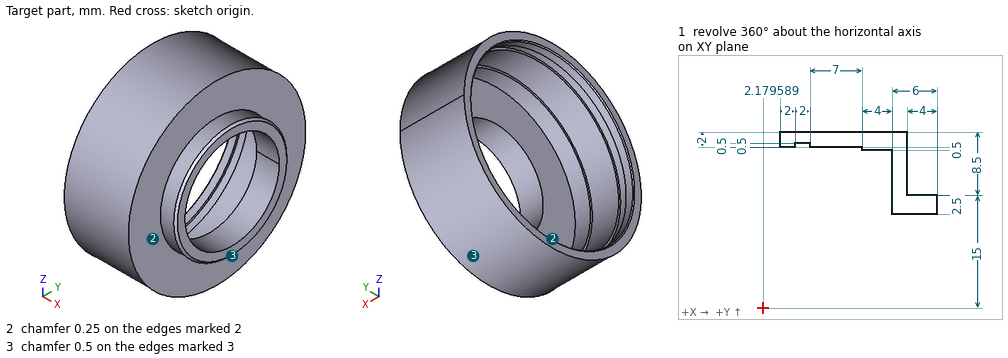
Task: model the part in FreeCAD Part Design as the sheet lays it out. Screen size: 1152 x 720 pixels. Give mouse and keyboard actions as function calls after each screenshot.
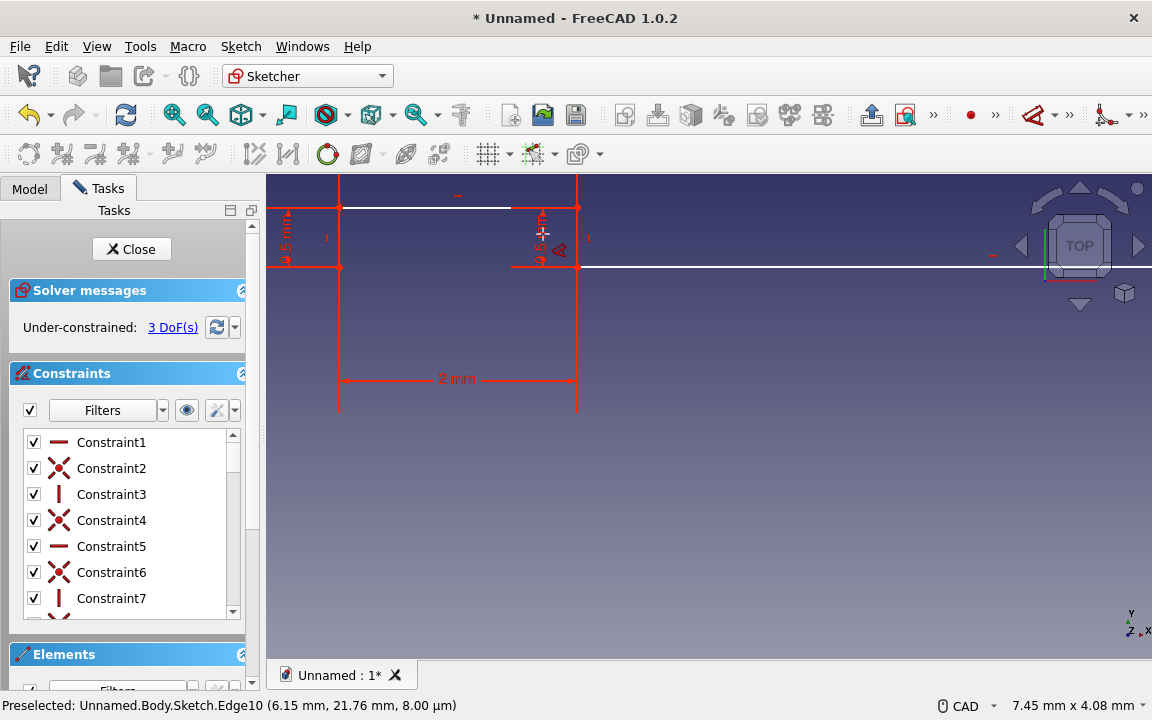
scroll(568, 292, down, 11)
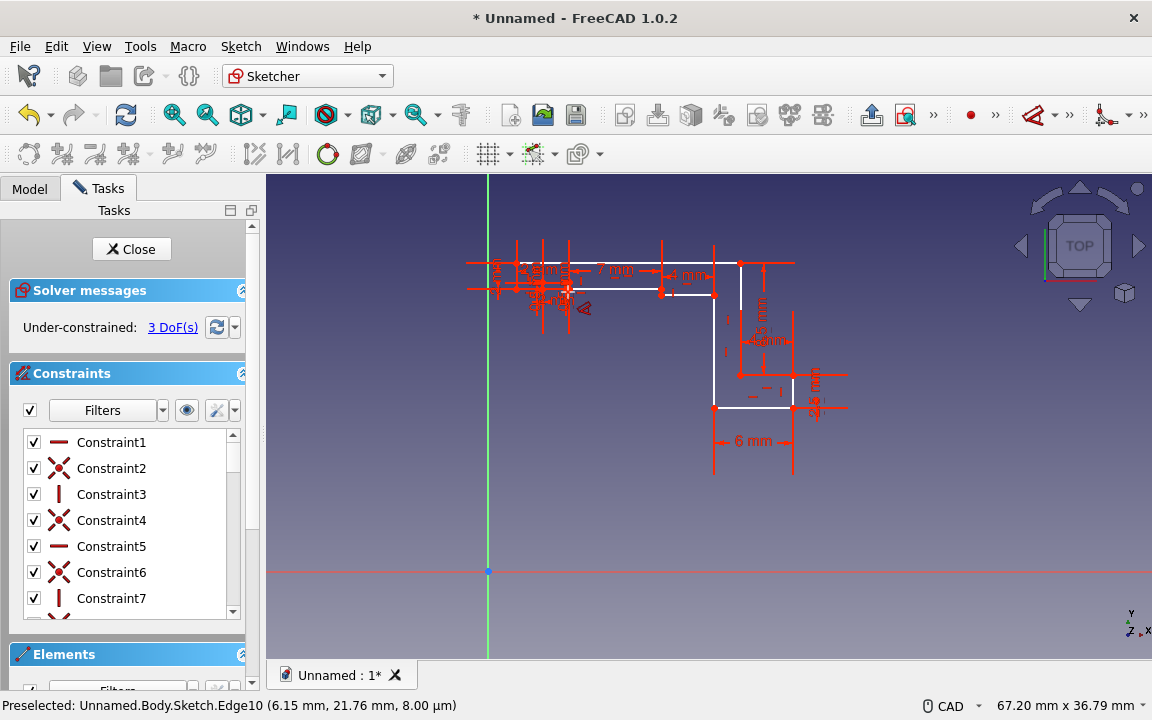
scroll(662, 291, up, 11)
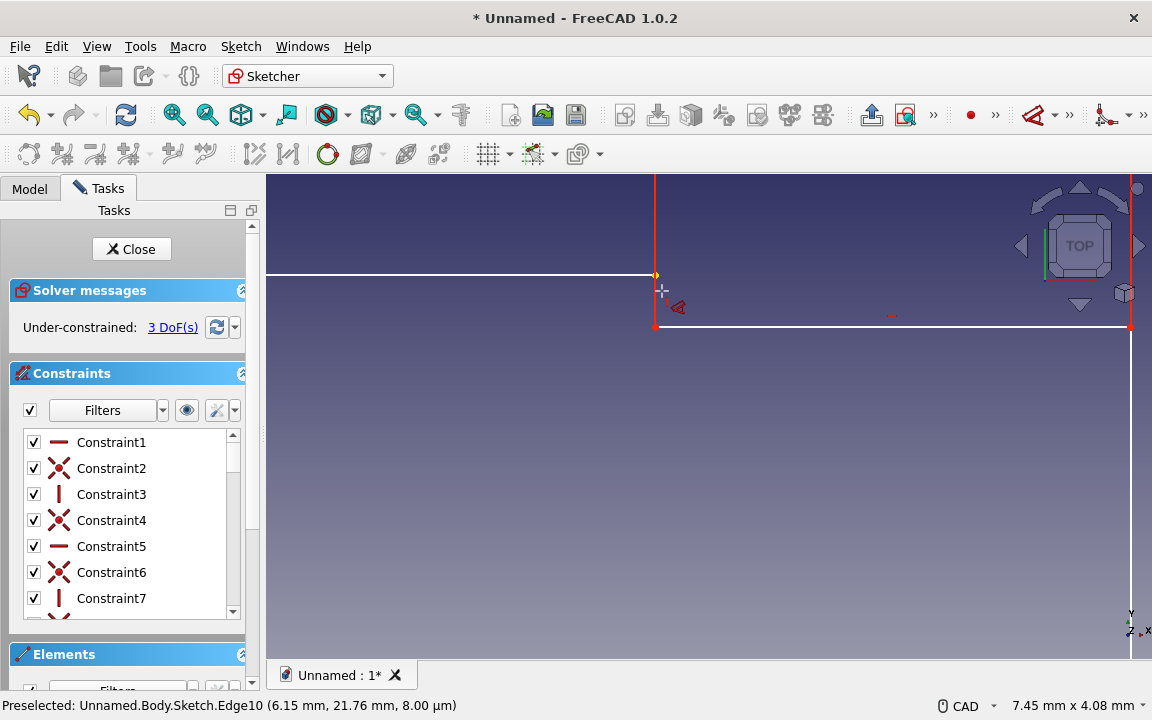
click(655, 291)
click(689, 301)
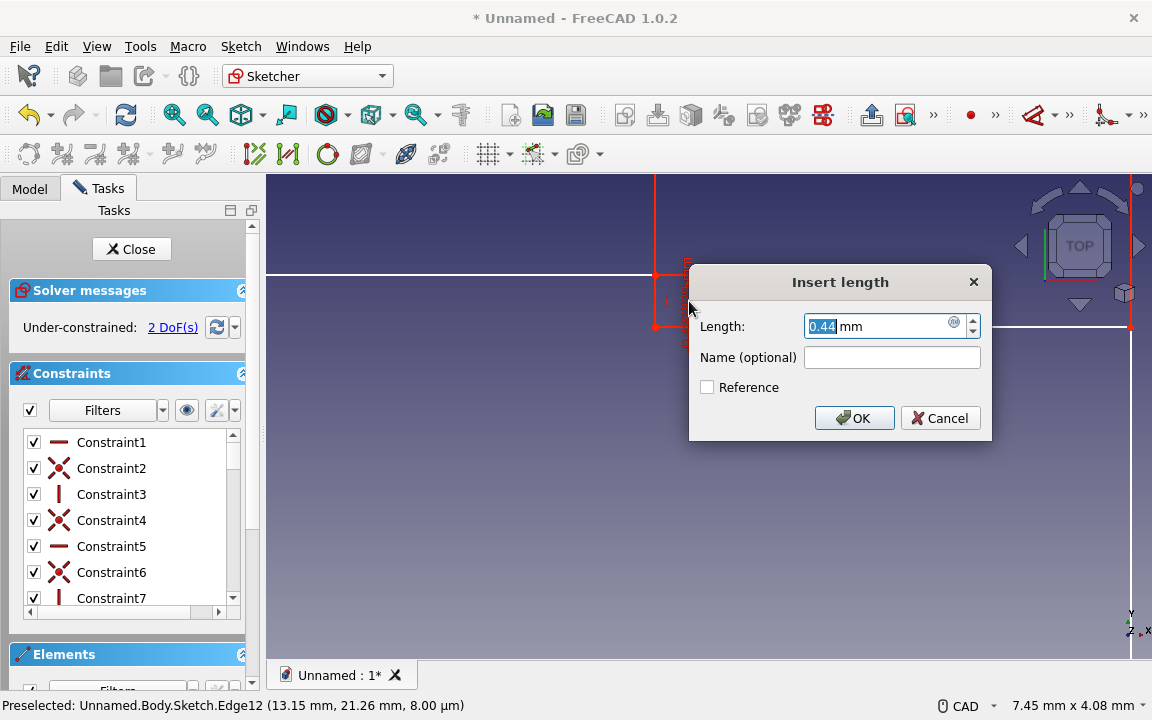
text(0.5)
key(Return)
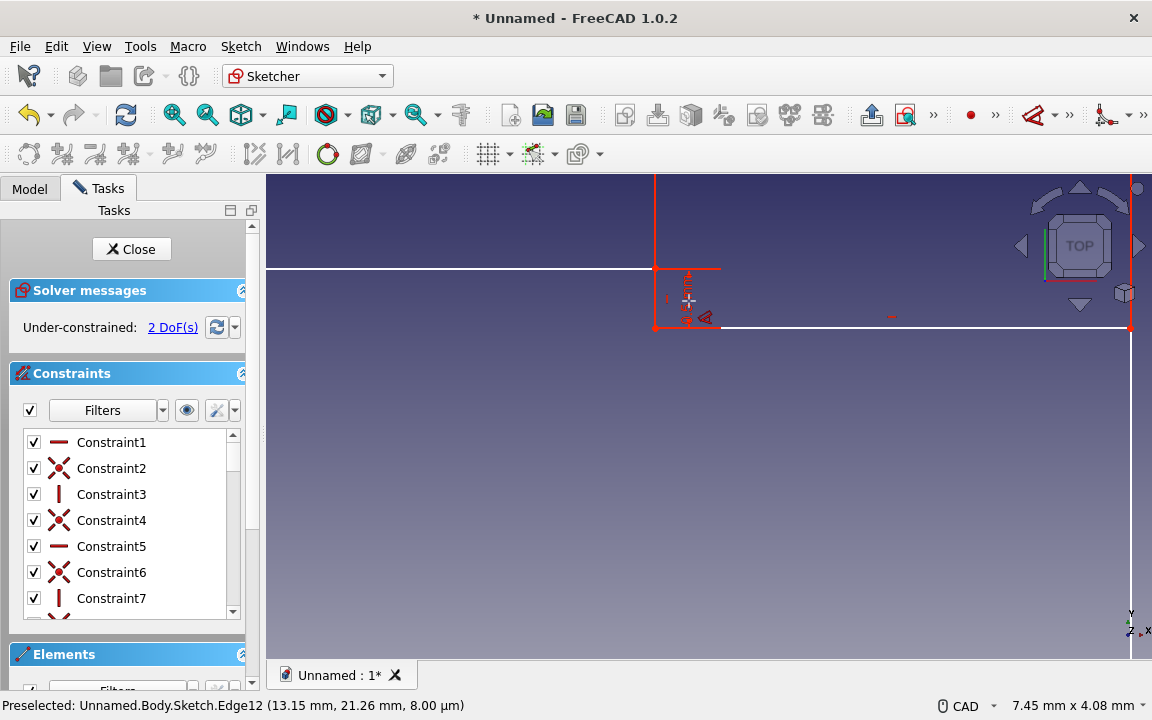
scroll(662, 291, down, 11)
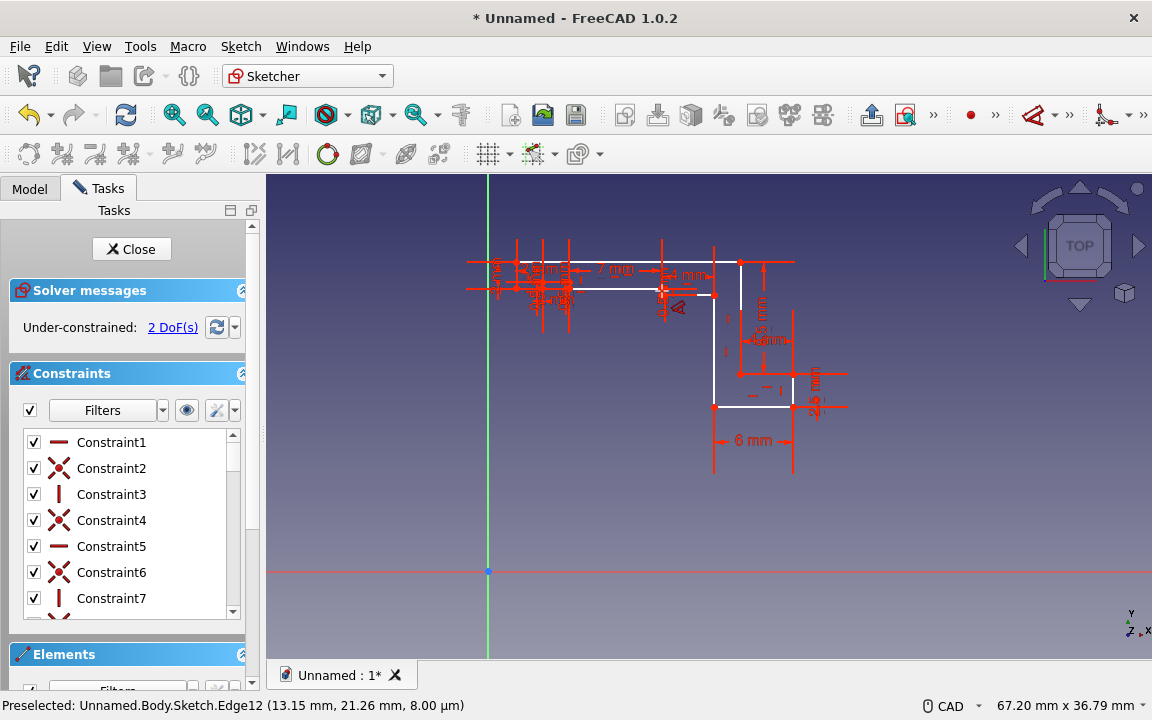
click(793, 374)
click(454, 473)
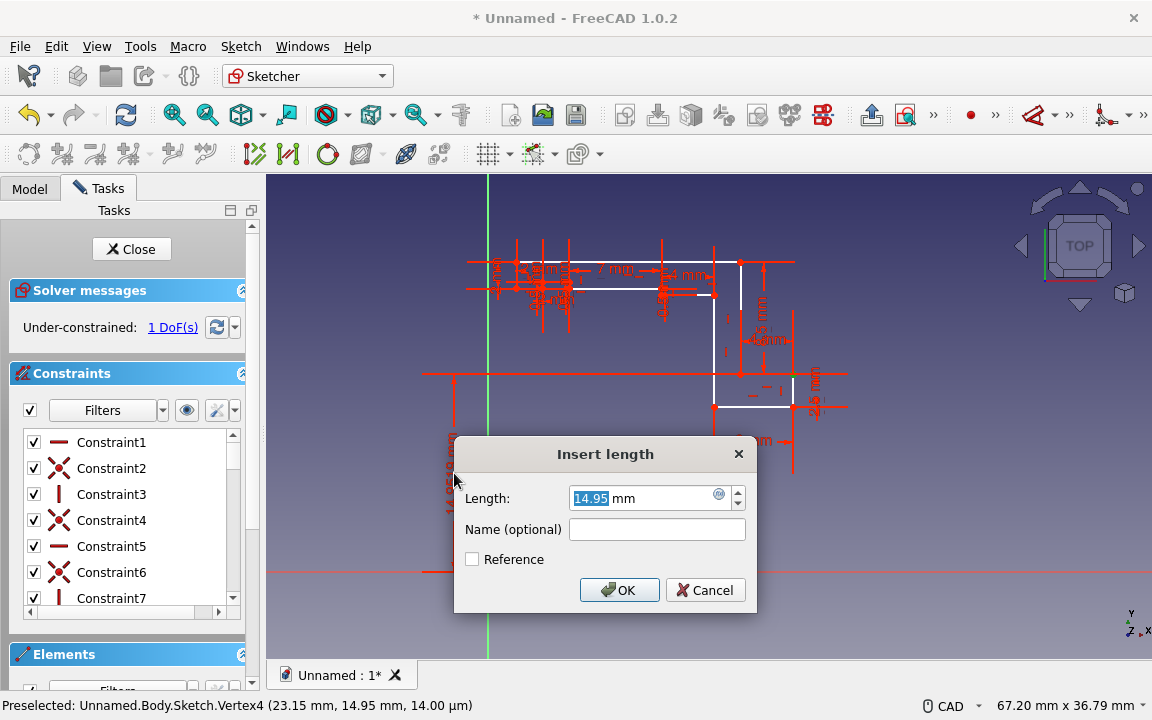
text(15)
key(Return)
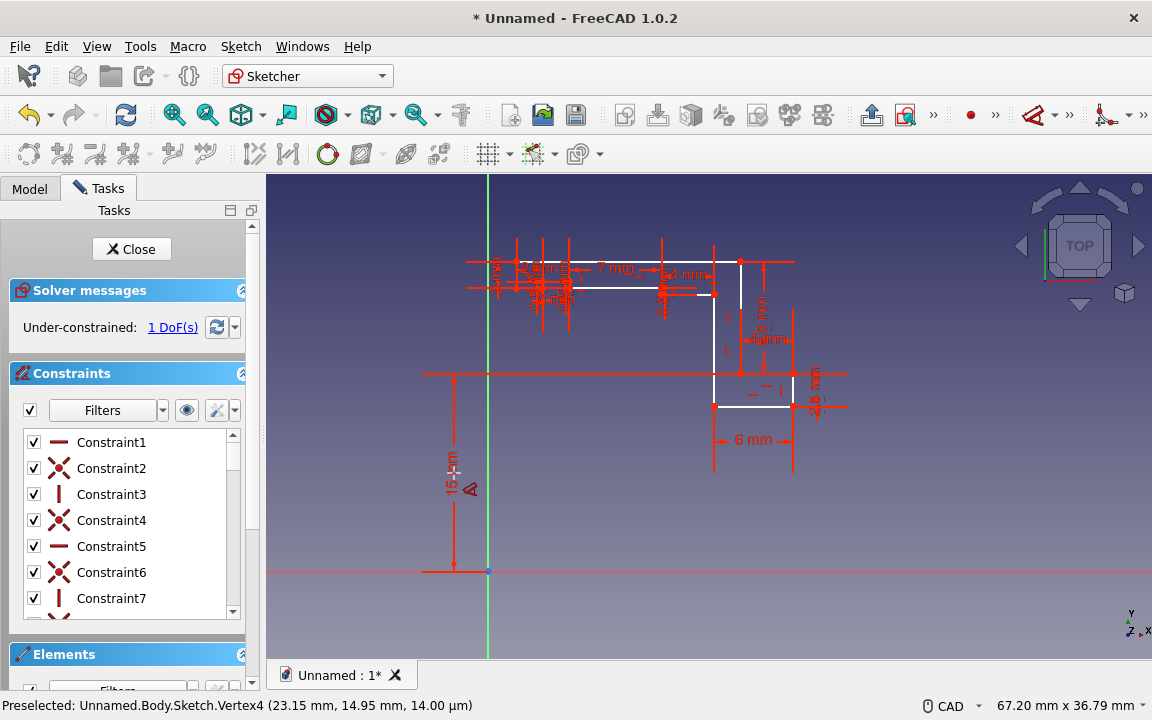
scroll(517, 262, up, 2)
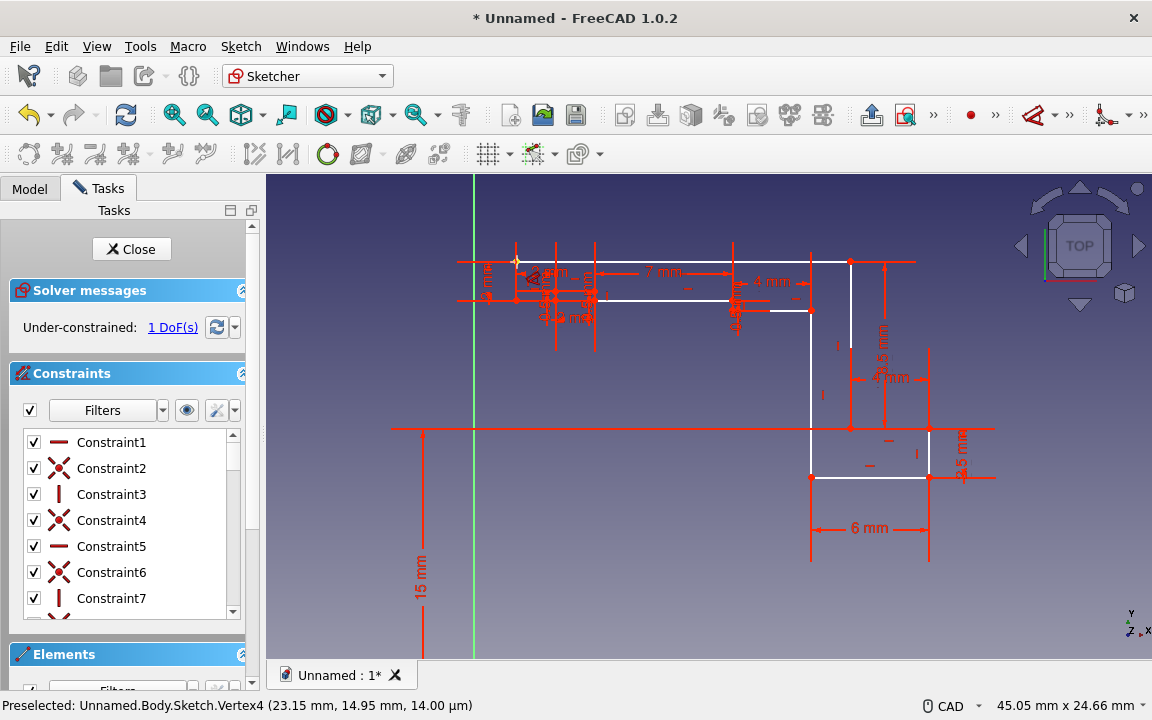
click(516, 262)
click(495, 228)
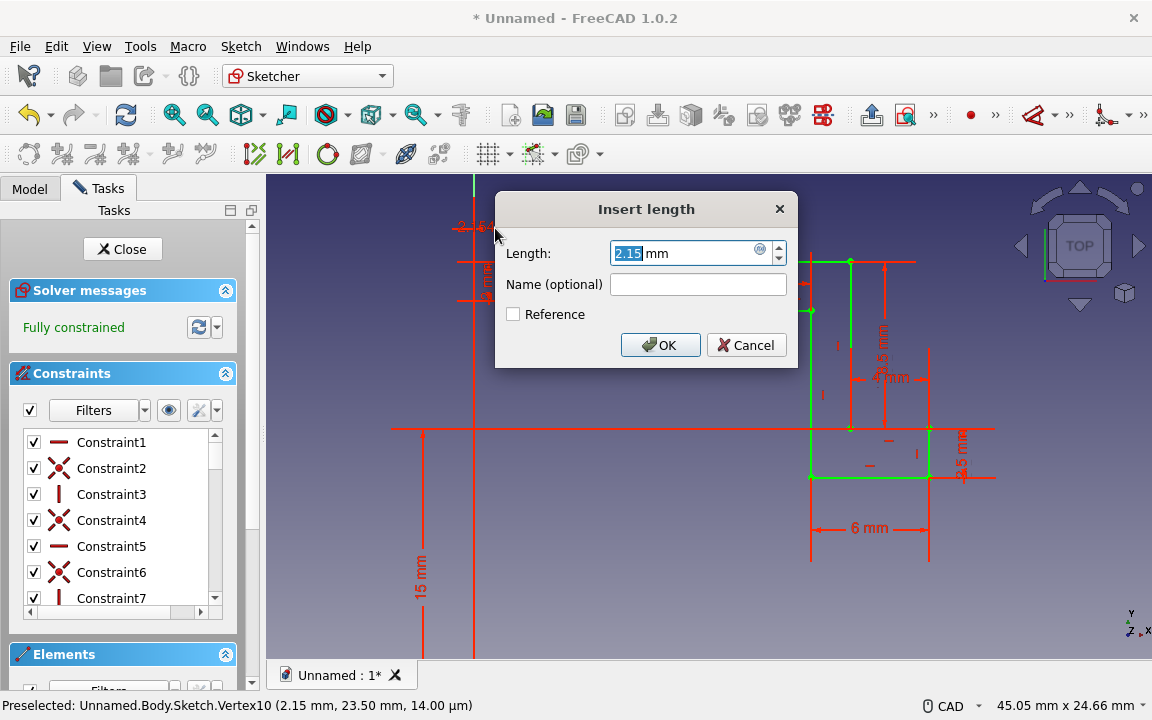
text(2.179589)
key(Return)
key(Escape)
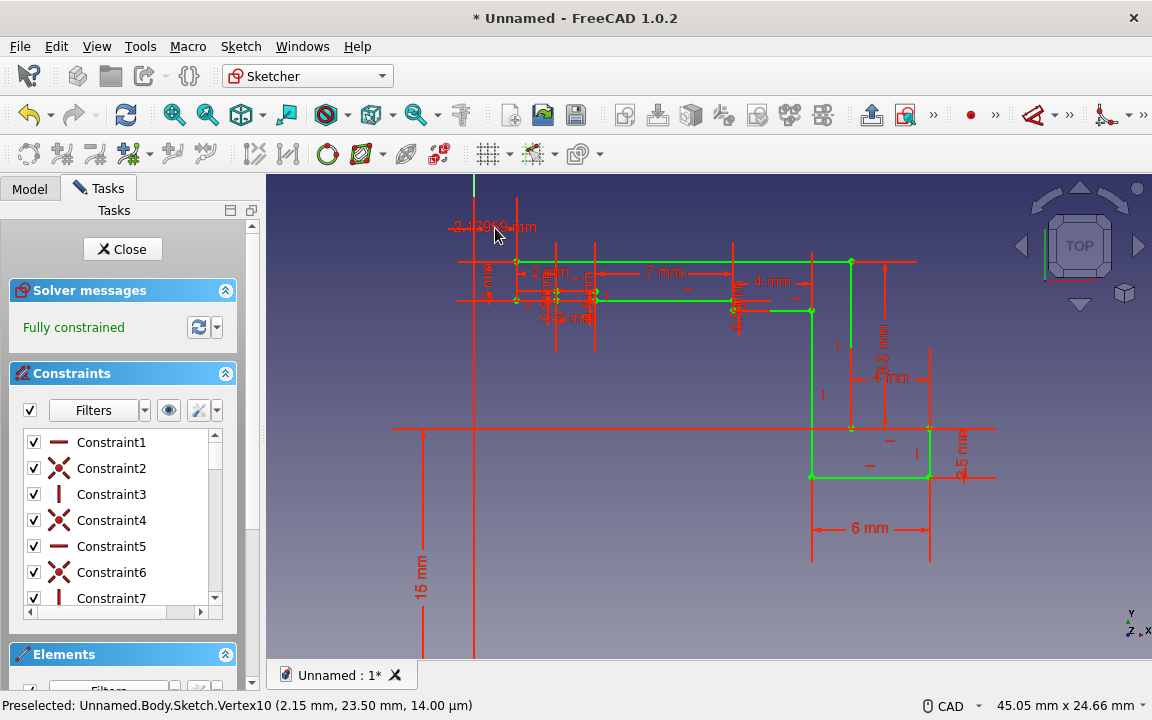
click(123, 249)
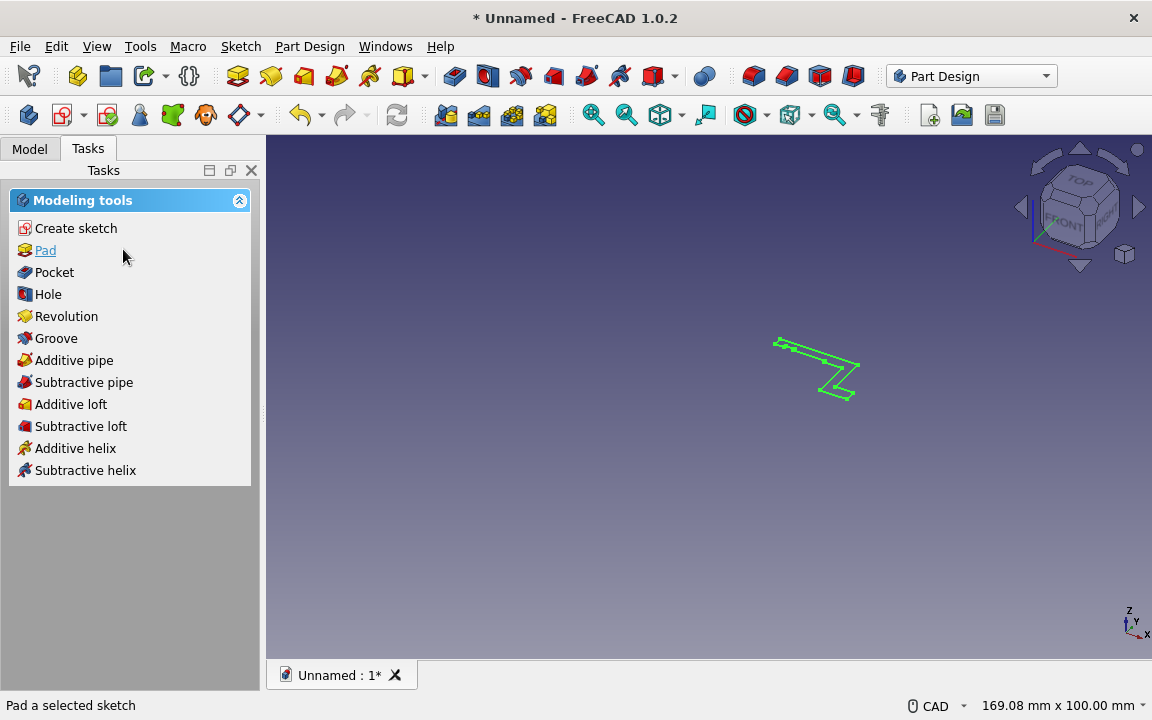
click(271, 76)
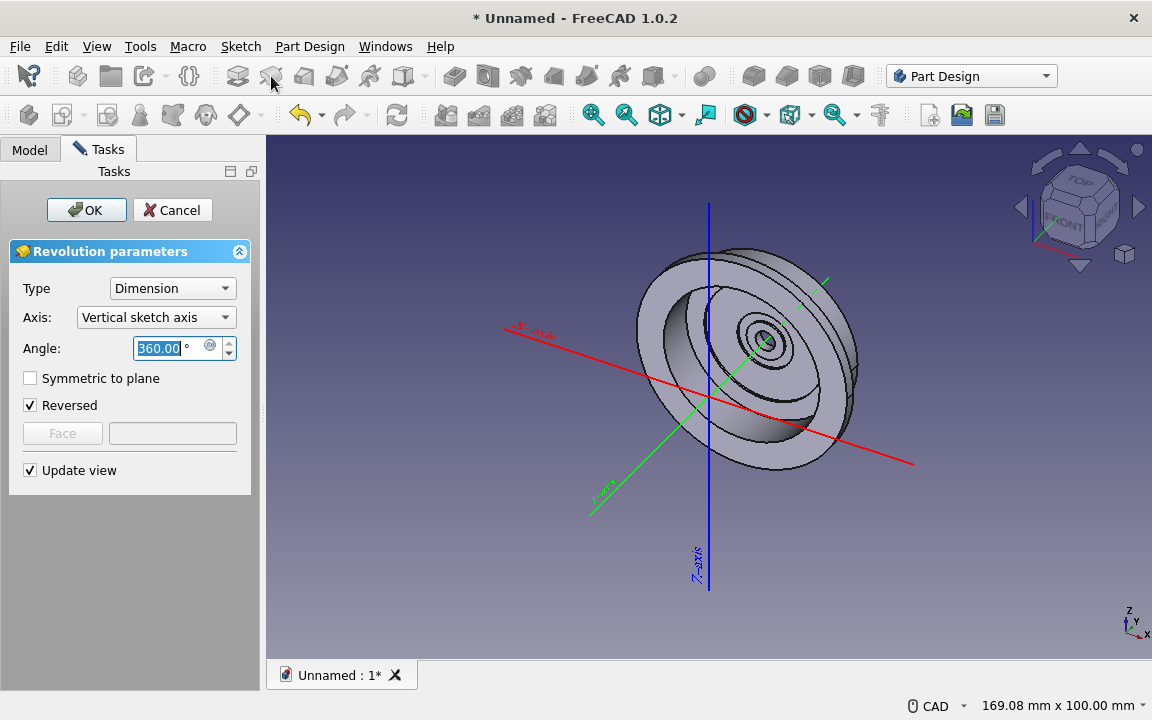
click(157, 318)